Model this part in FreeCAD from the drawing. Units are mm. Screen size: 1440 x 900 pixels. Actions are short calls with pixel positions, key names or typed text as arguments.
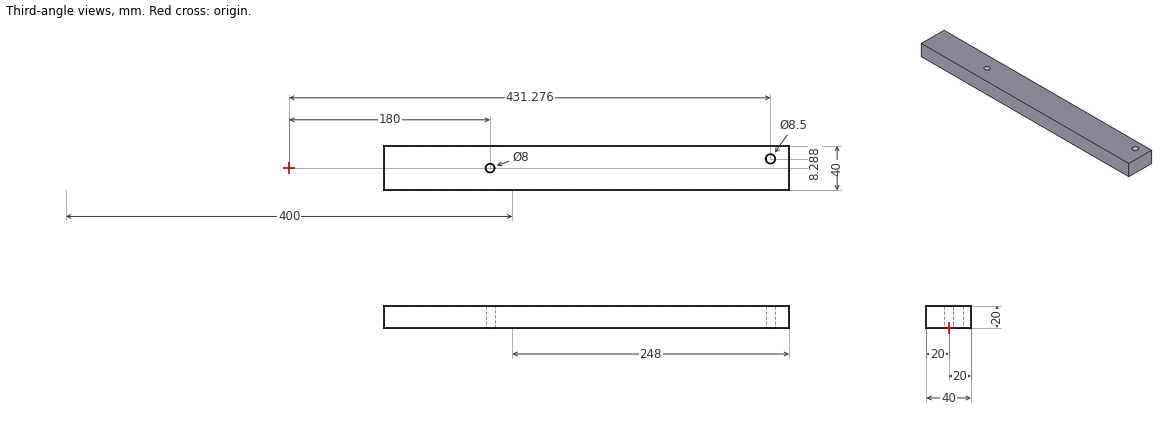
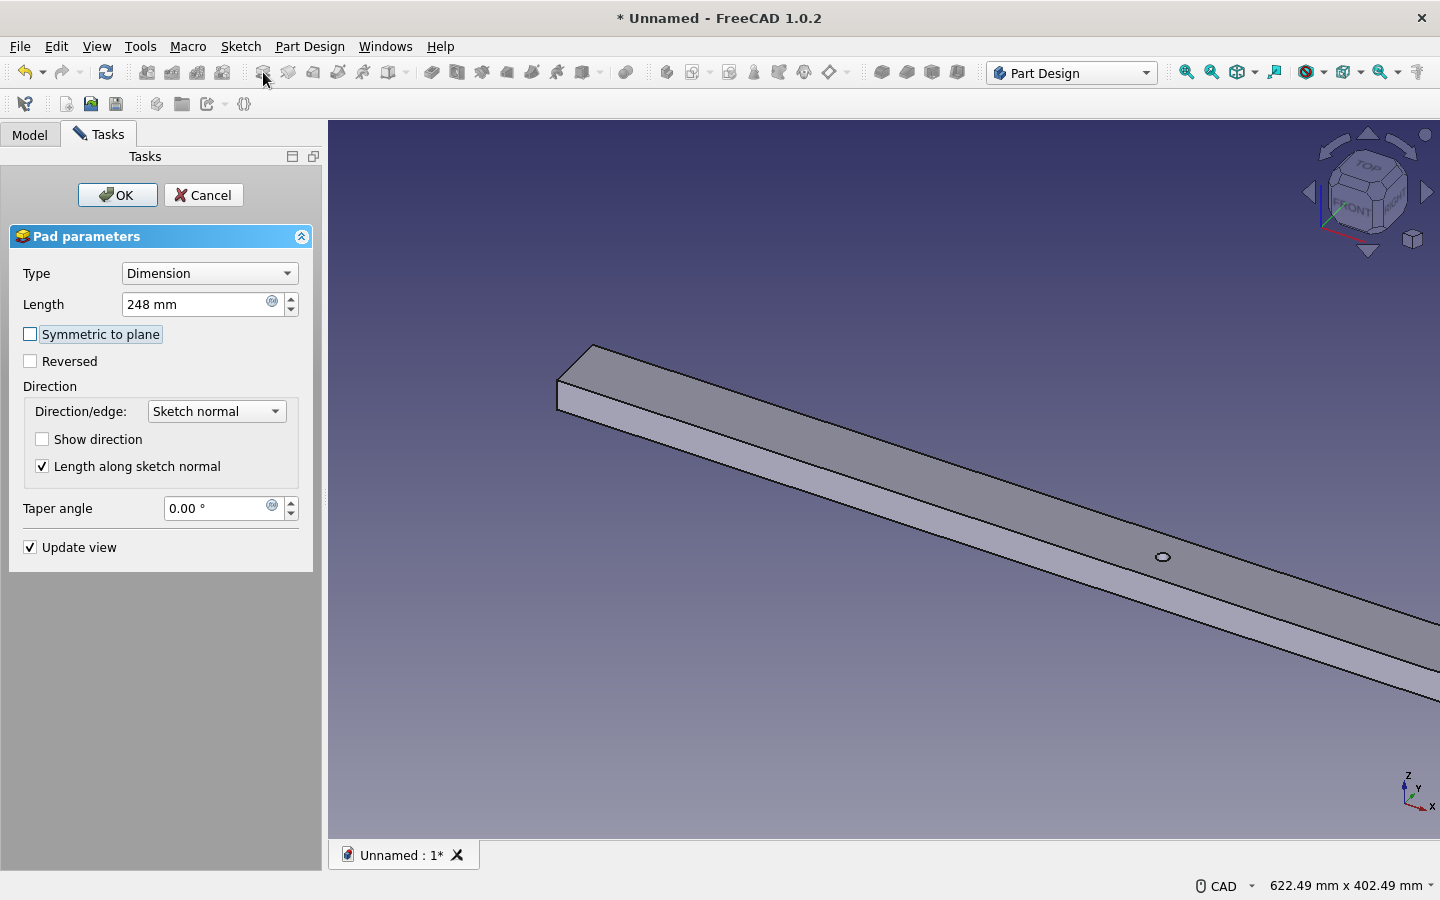
click(118, 195)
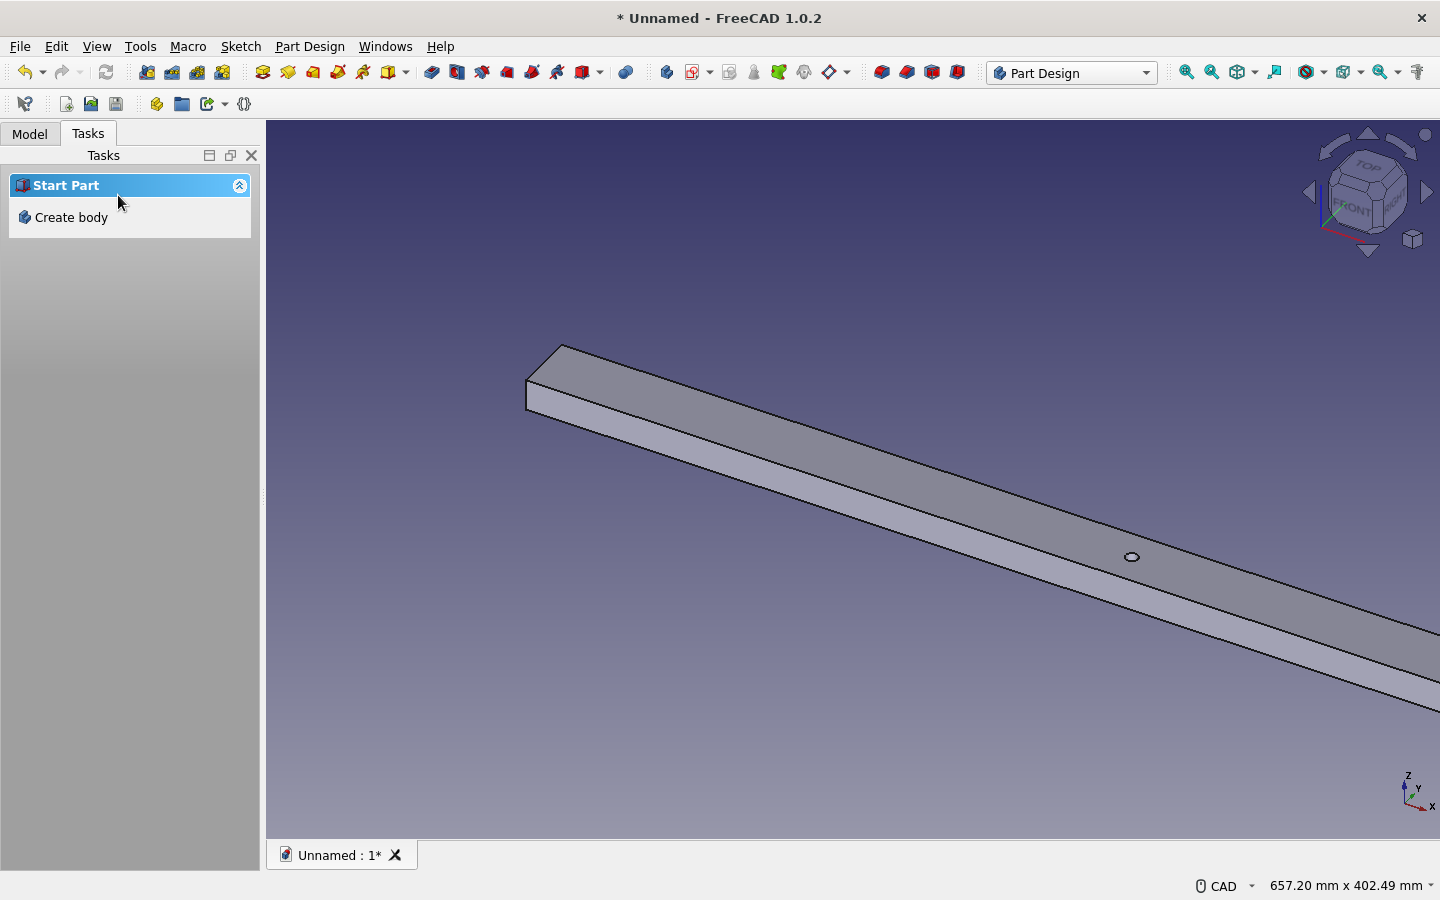
click(1187, 72)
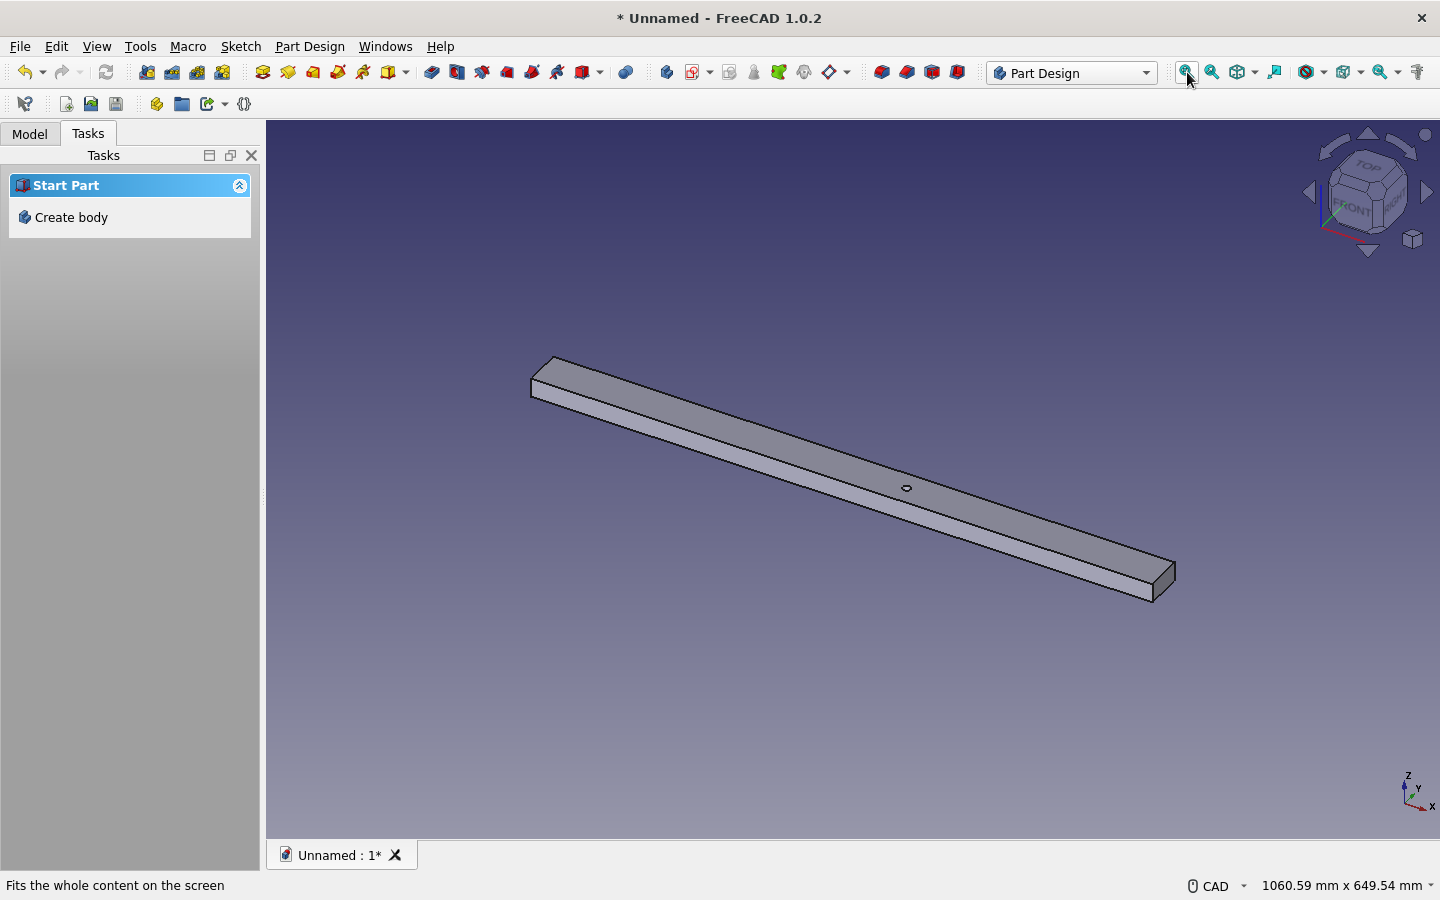
click(1119, 558)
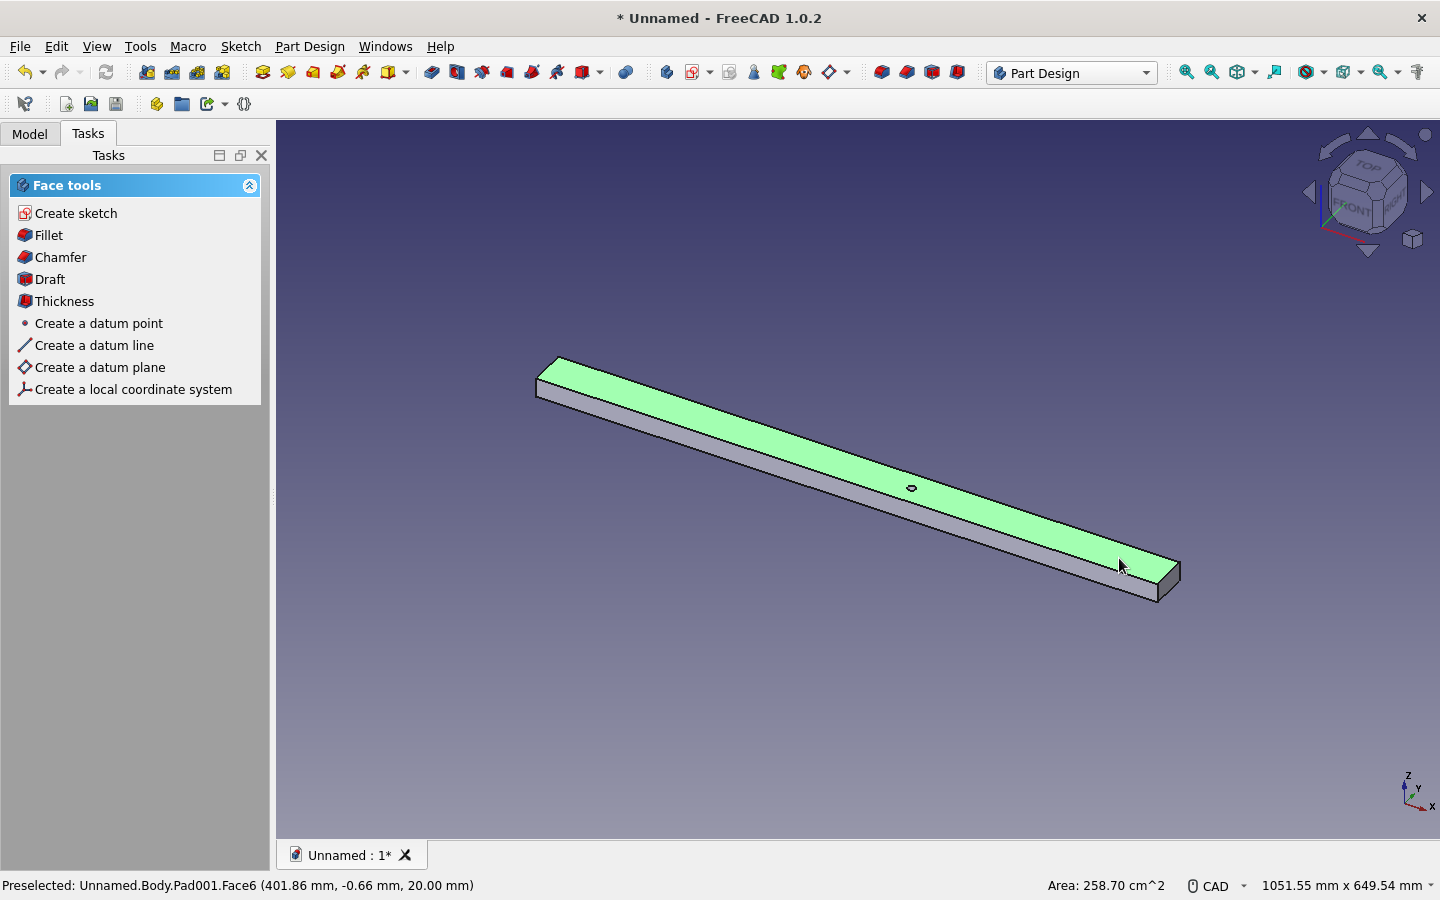
click(692, 72)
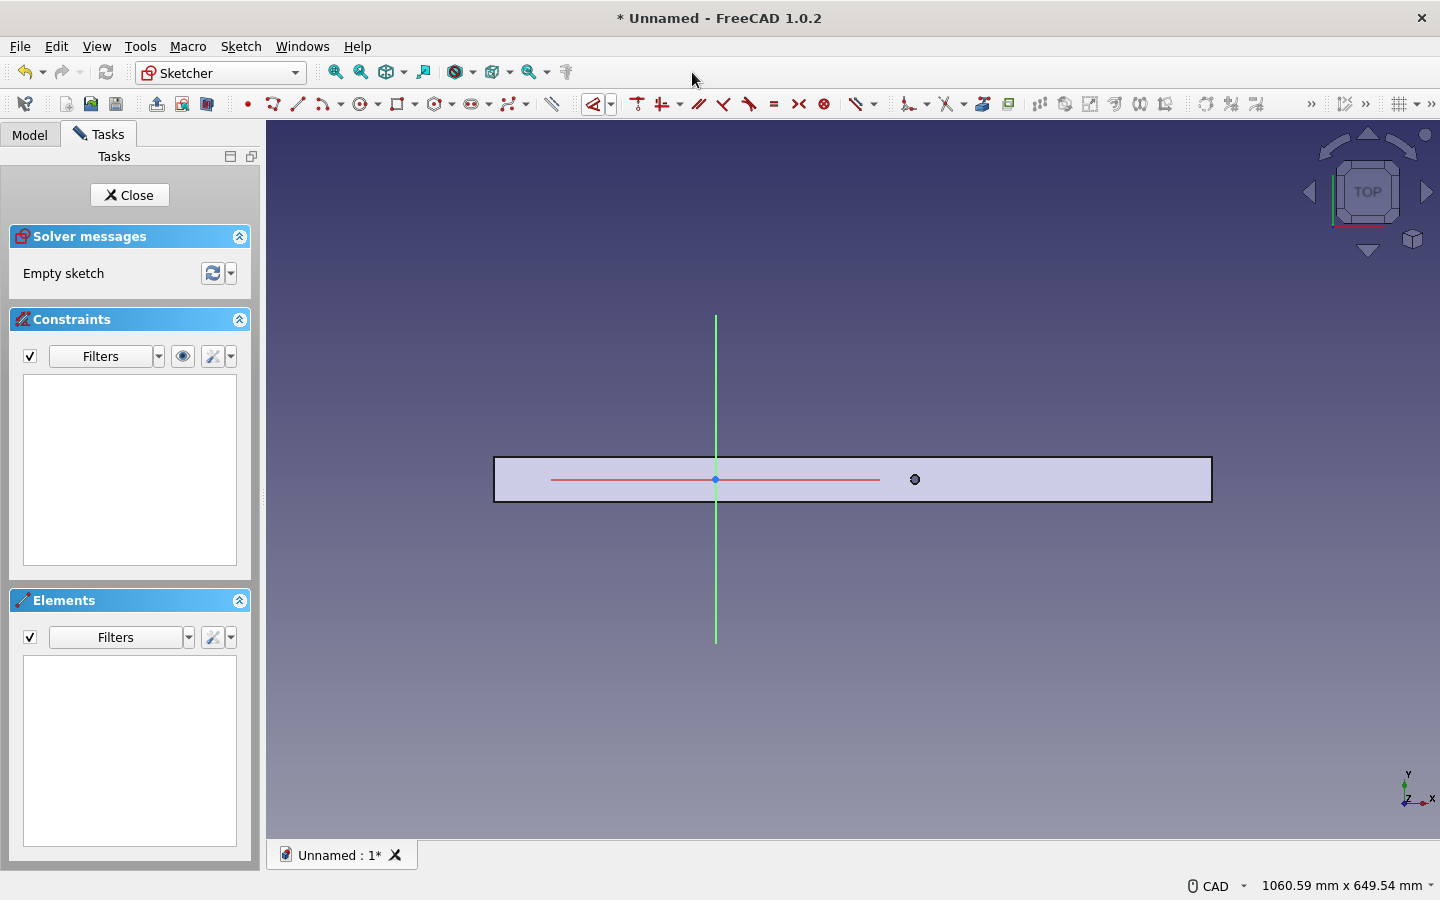
scroll(1215, 470, up, 15)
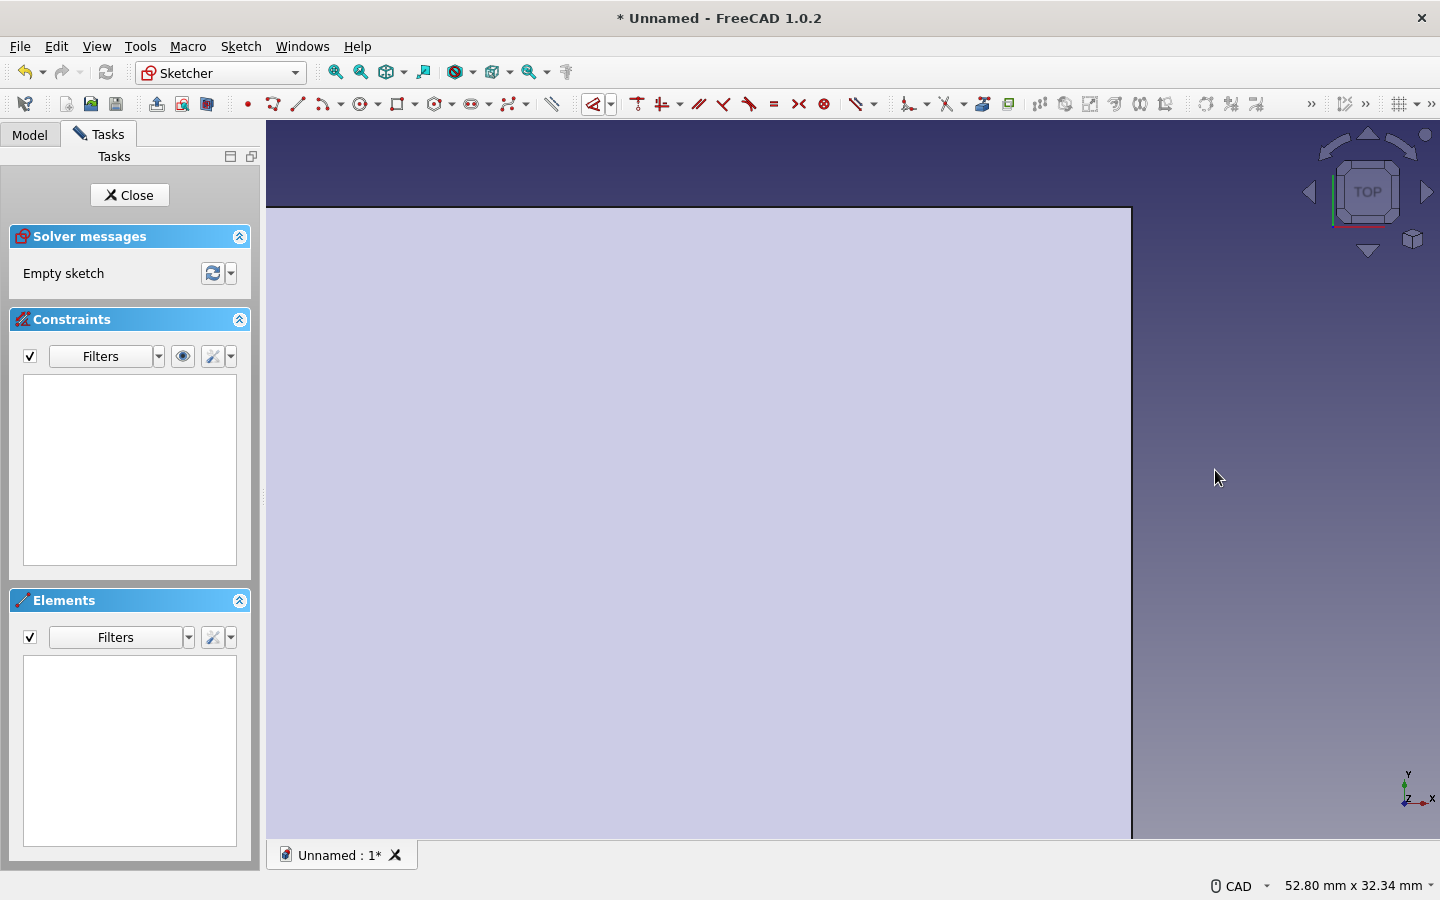
scroll(746, 460, up, 5)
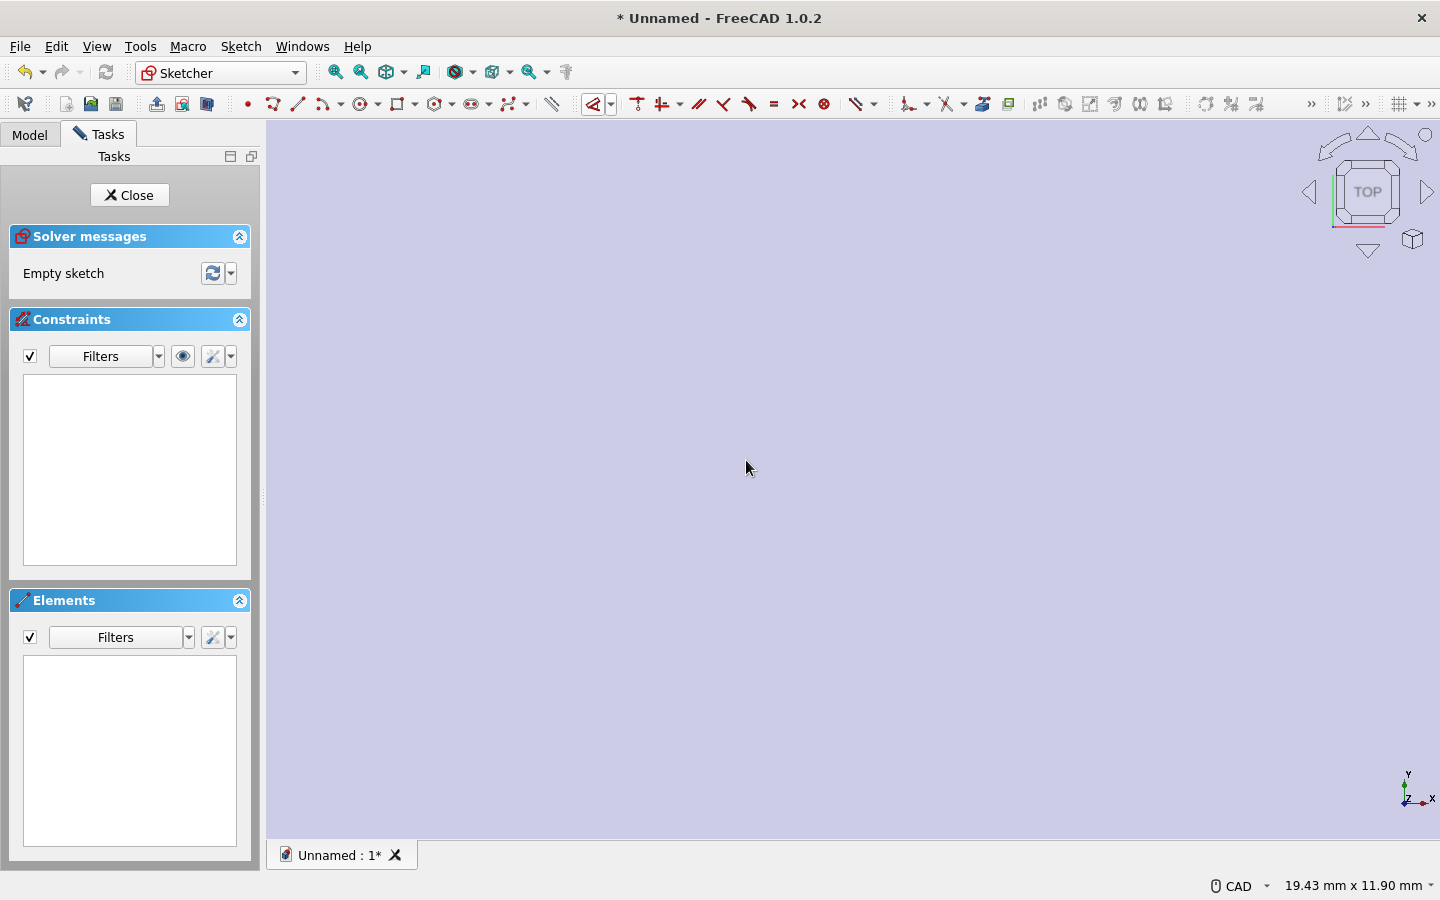
click(360, 104)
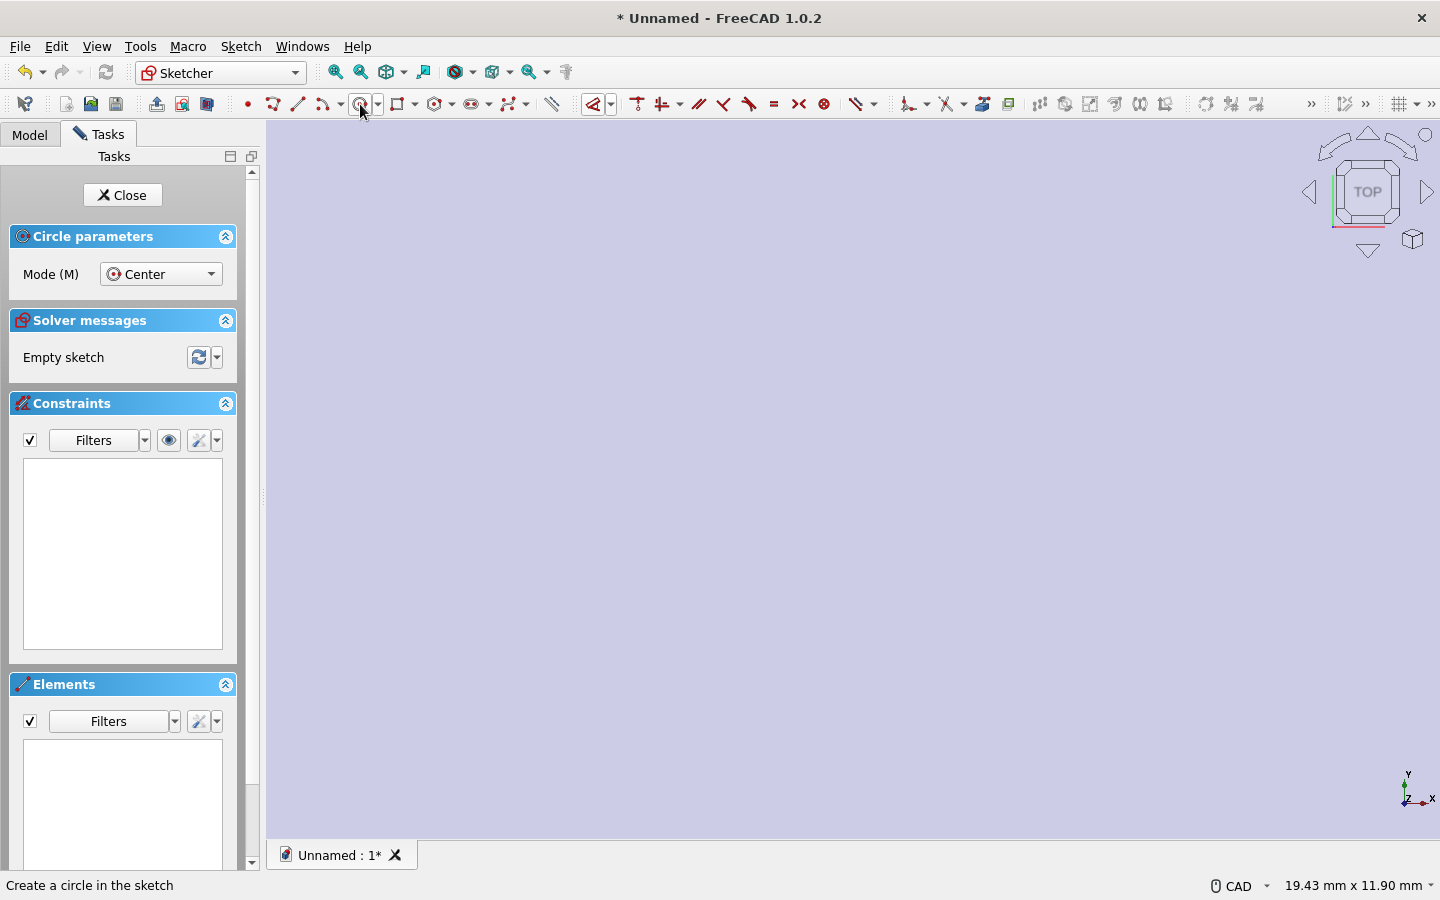
click(784, 479)
click(966, 297)
key(Escape)